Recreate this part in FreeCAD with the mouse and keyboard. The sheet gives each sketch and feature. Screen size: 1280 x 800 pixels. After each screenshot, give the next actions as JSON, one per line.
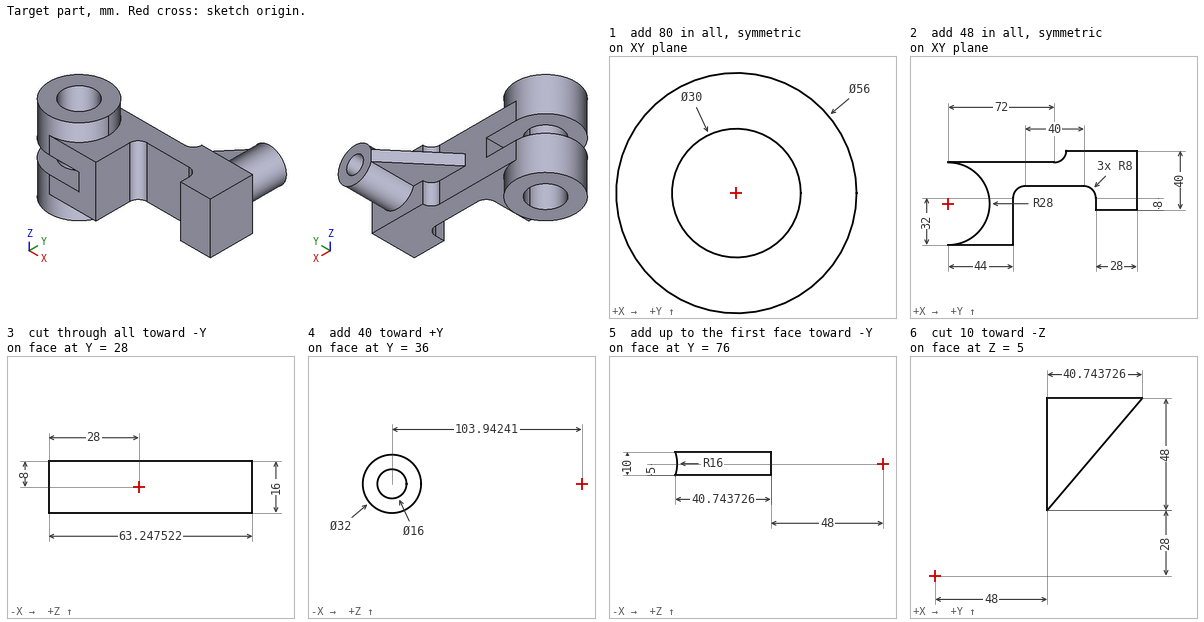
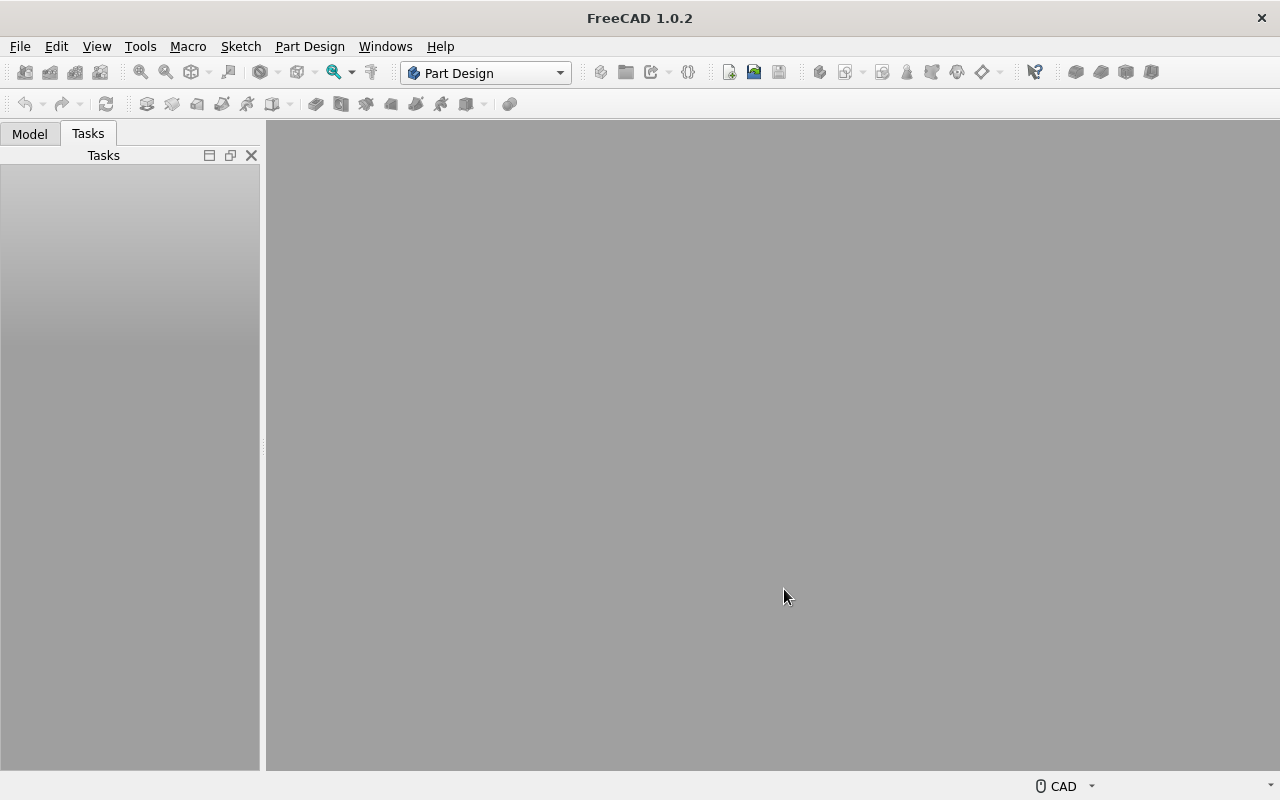
{"action": "left_click", "coordinate": [729, 72]}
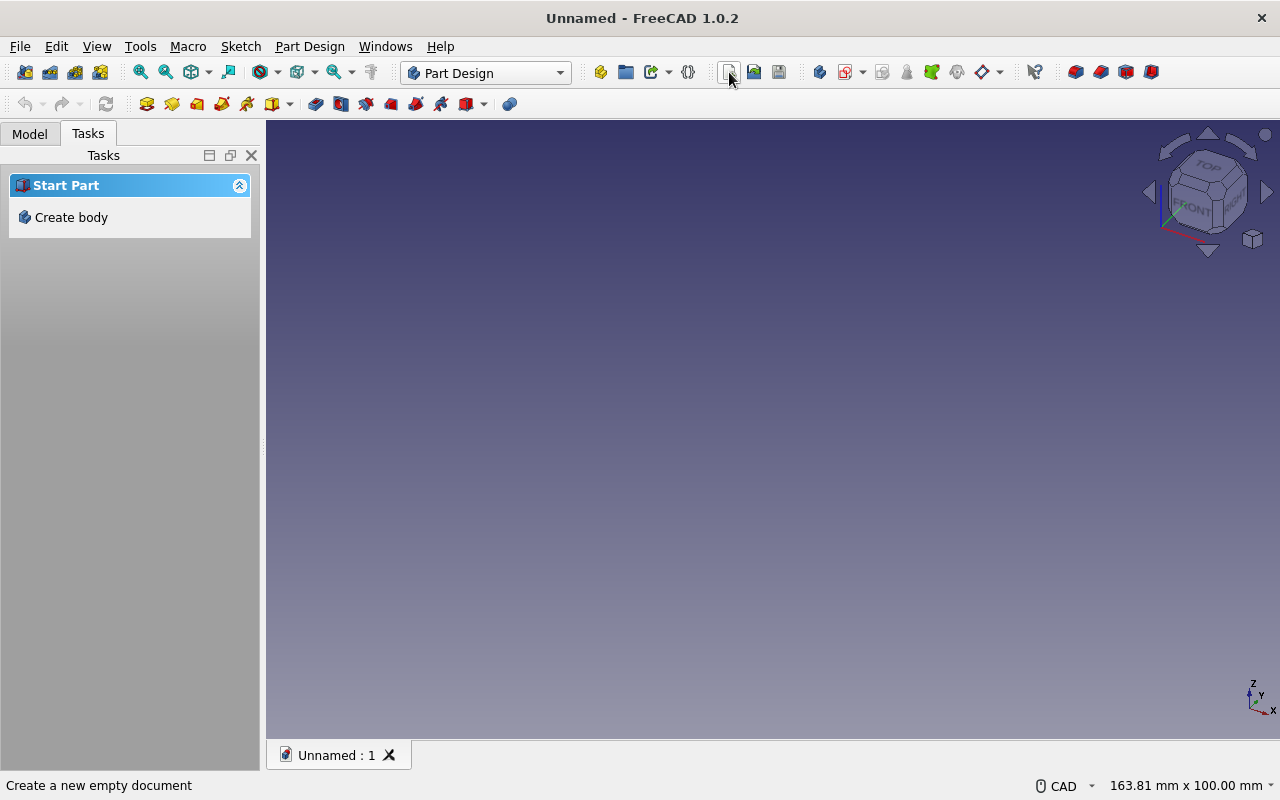
{"action": "left_click", "coordinate": [844, 72]}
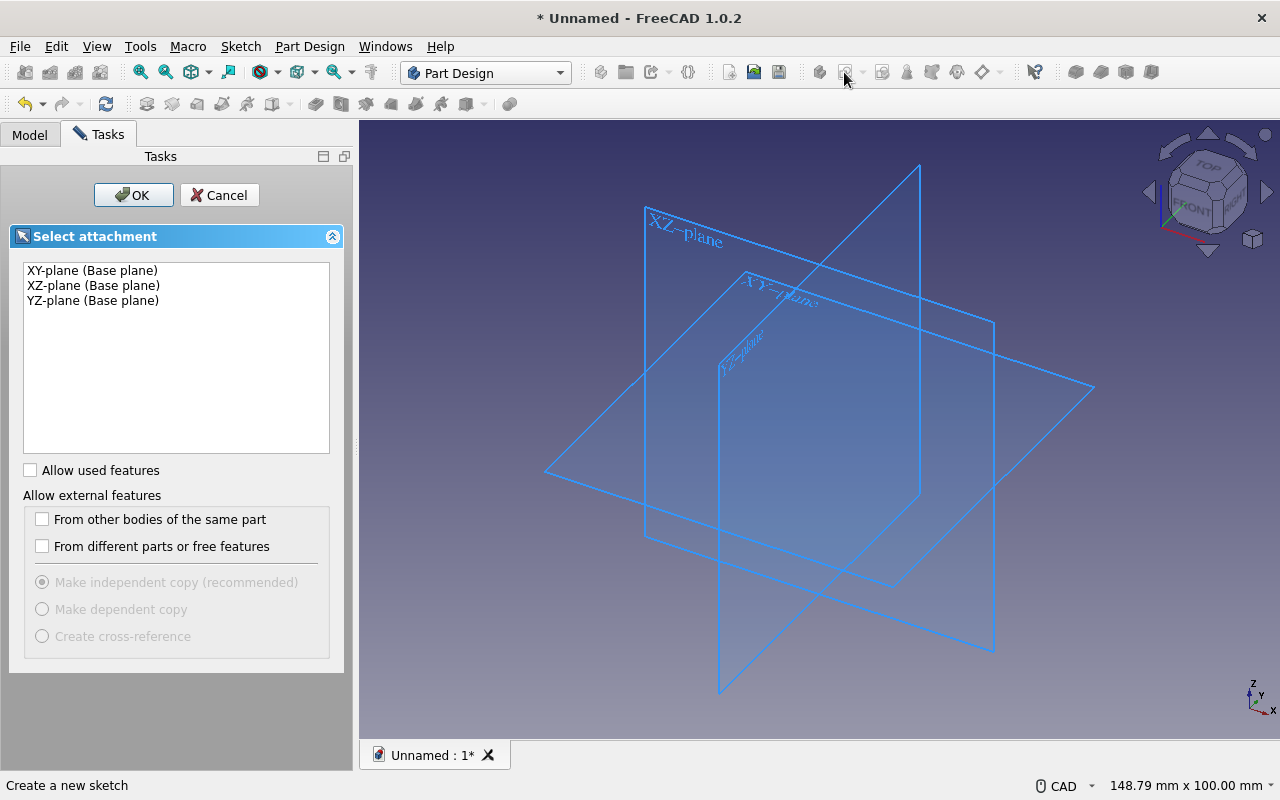
{"action": "left_click", "coordinate": [84, 270]}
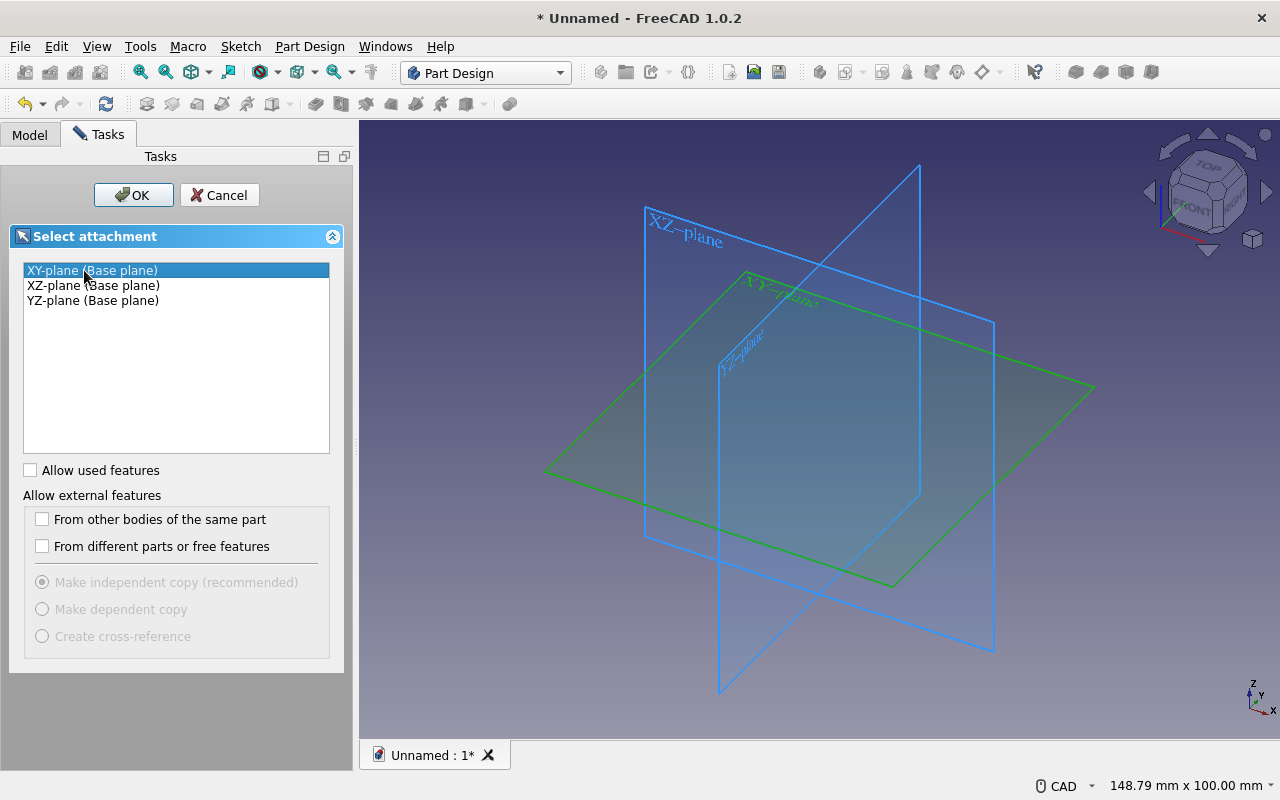
{"action": "left_click", "coordinate": [134, 195]}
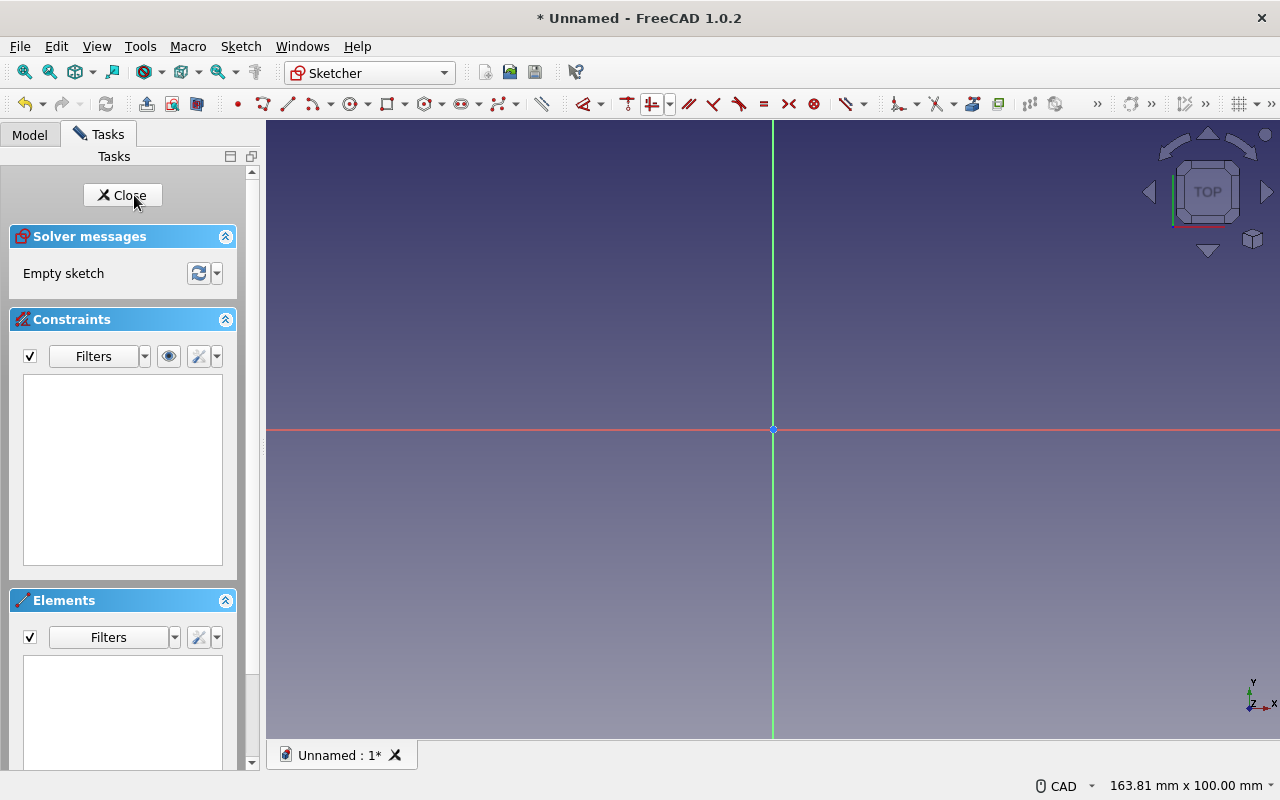
{"action": "key", "text": "g c"}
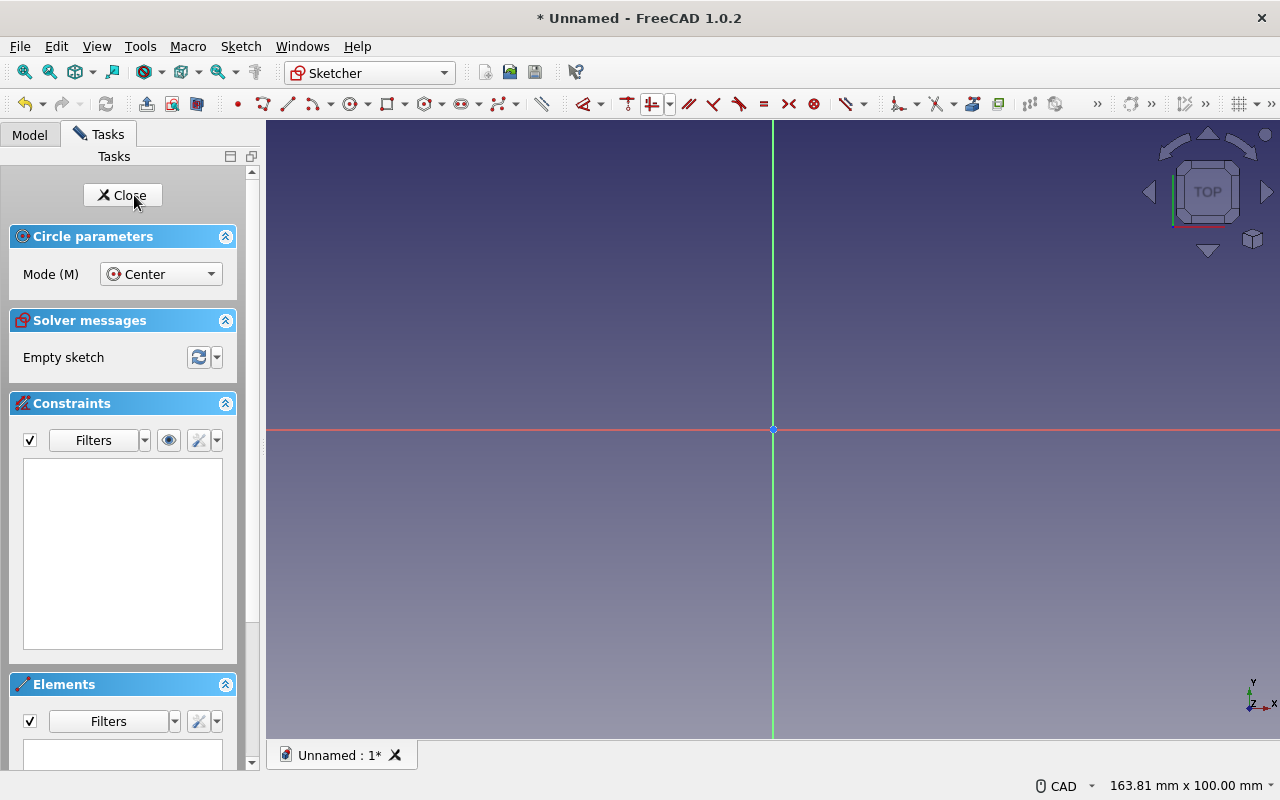
{"action": "left_click", "coordinate": [773, 430]}
{"action": "mouse_move", "coordinate": [896, 307]}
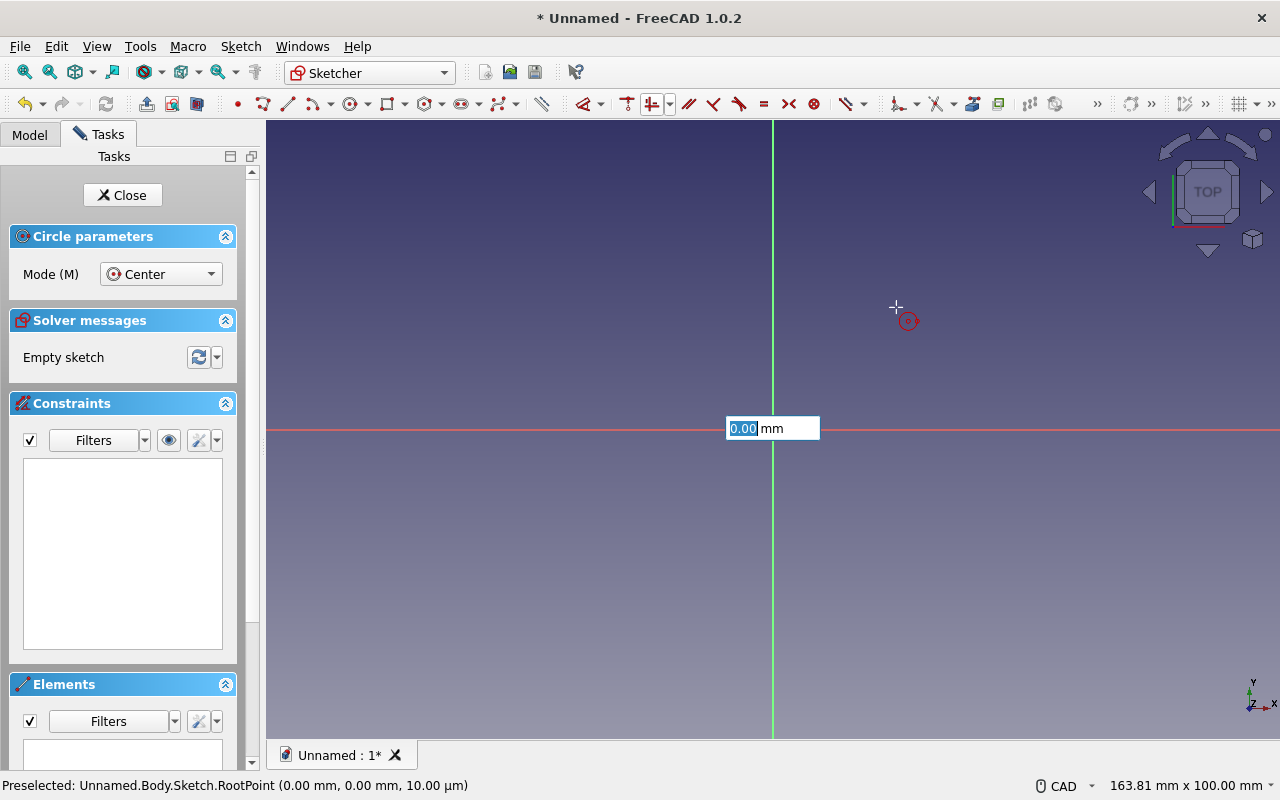
{"action": "type", "text": "56"}
{"action": "key", "text": "Return"}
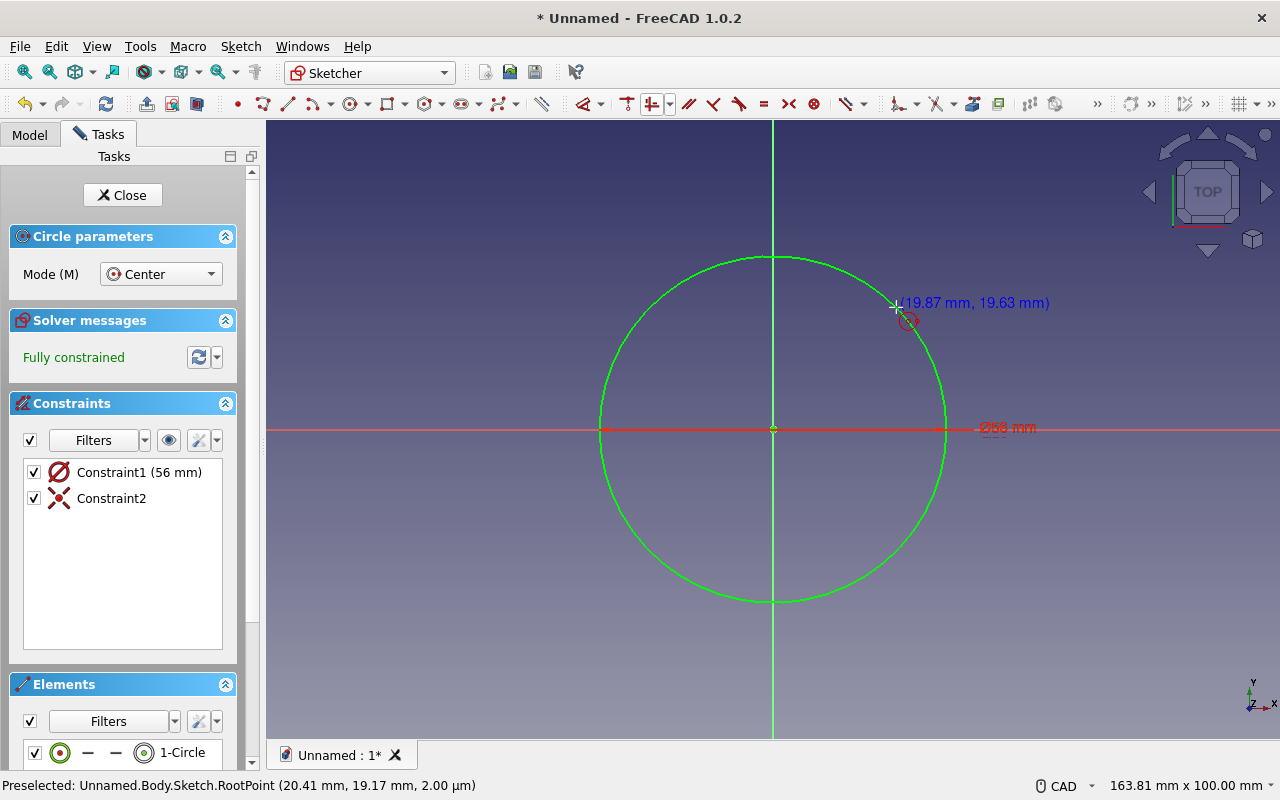
{"action": "left_click", "coordinate": [773, 430]}
{"action": "mouse_move", "coordinate": [839, 364]}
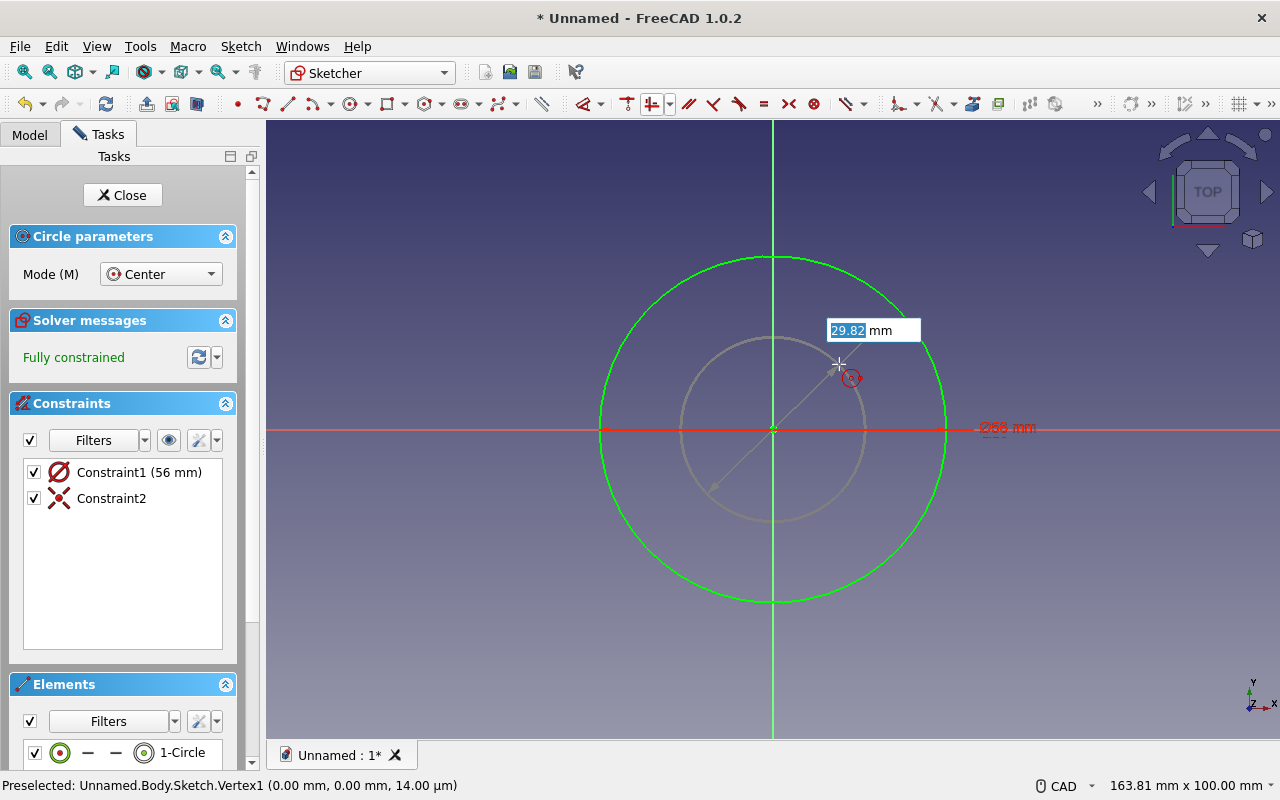
{"action": "type", "text": "30"}
{"action": "key", "text": "Return"}
{"action": "key", "text": "Escape"}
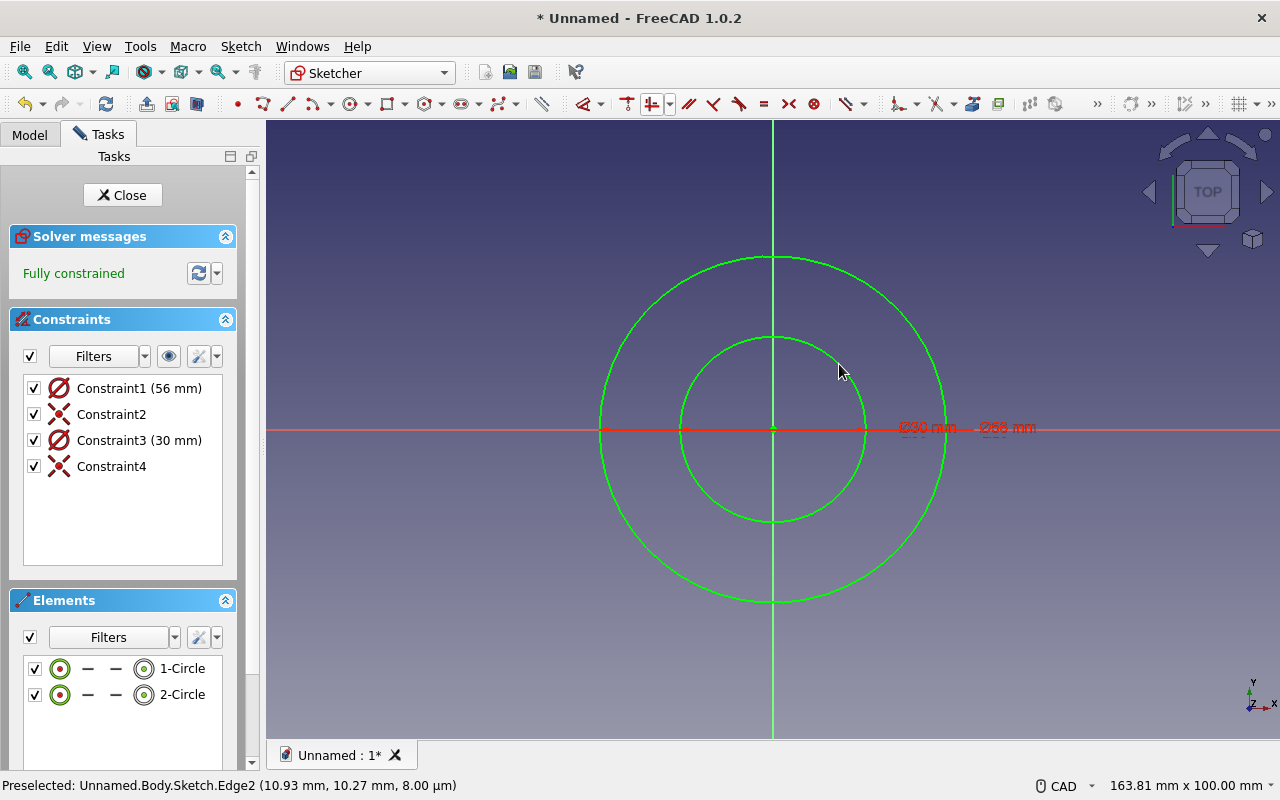
{"action": "left_click", "coordinate": [123, 195]}